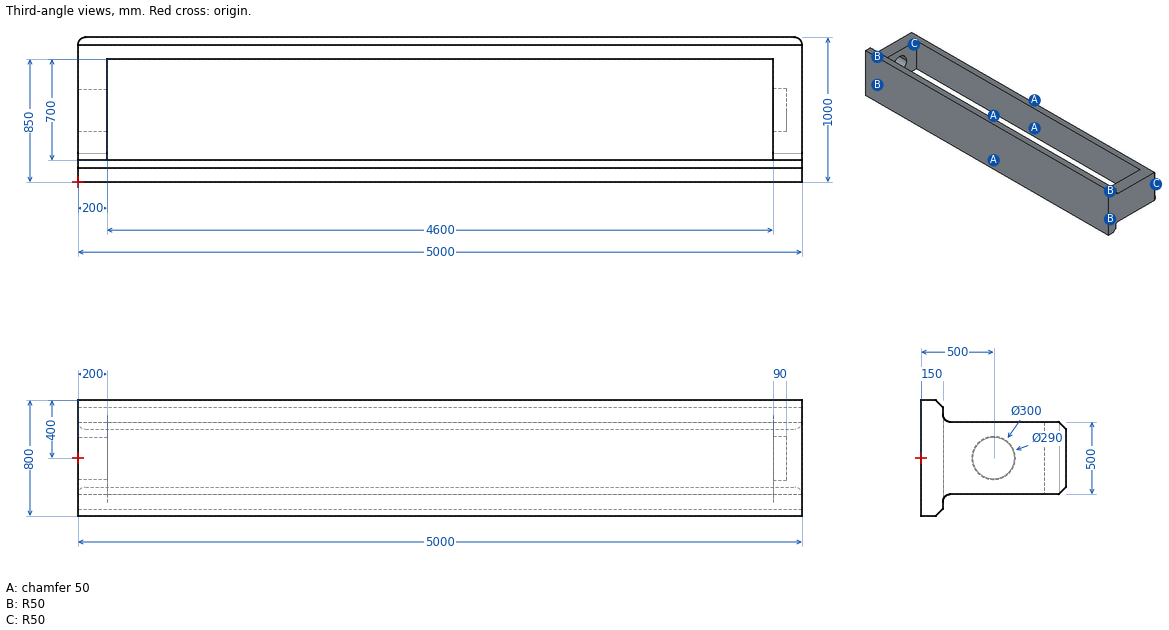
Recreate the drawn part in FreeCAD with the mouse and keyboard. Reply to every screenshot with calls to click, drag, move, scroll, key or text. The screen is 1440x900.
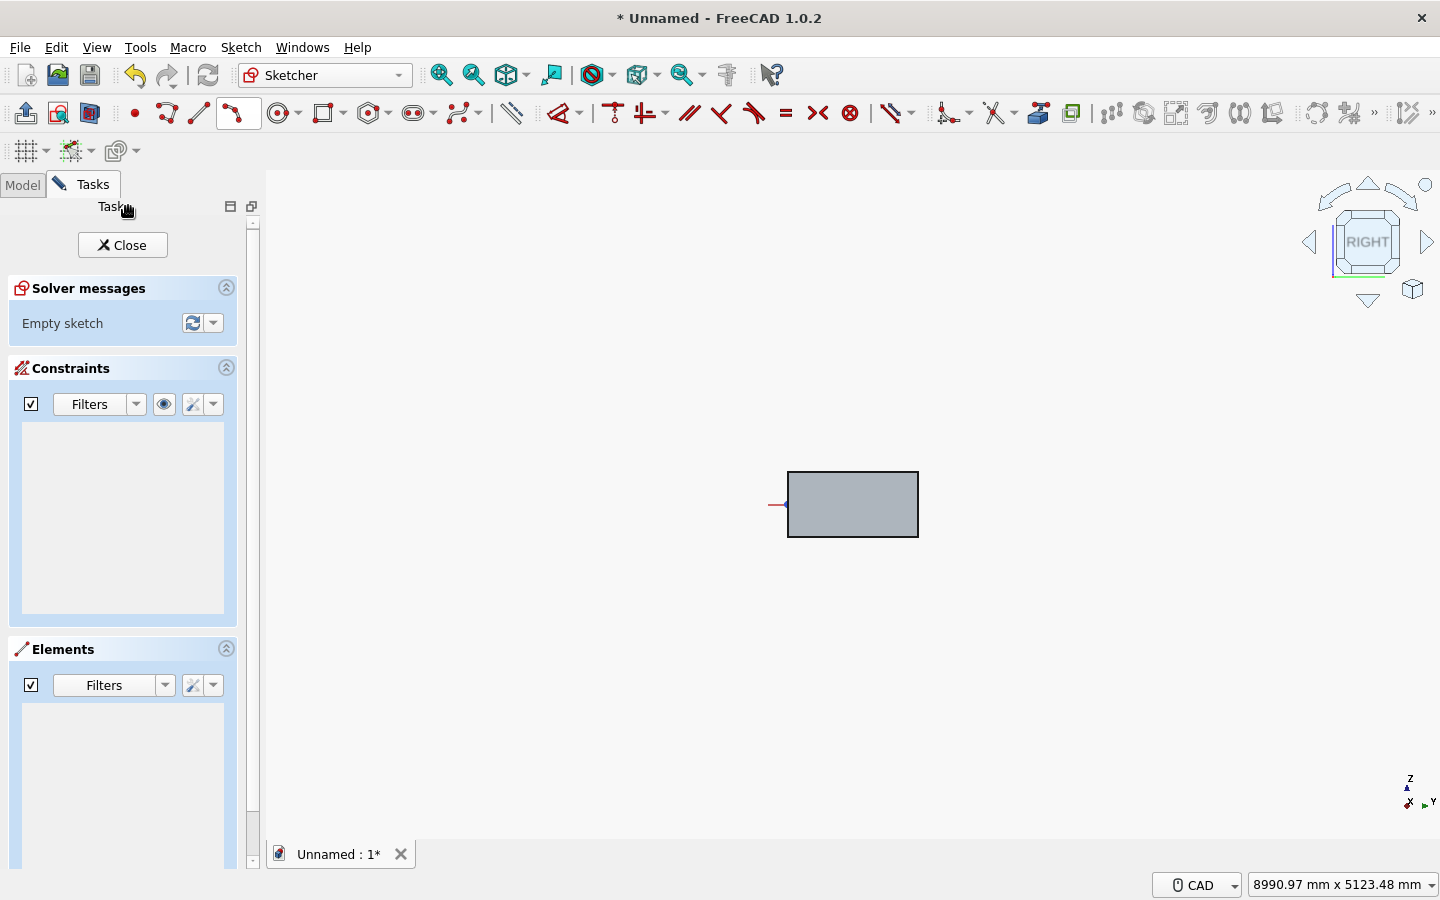
key(q)
key(s)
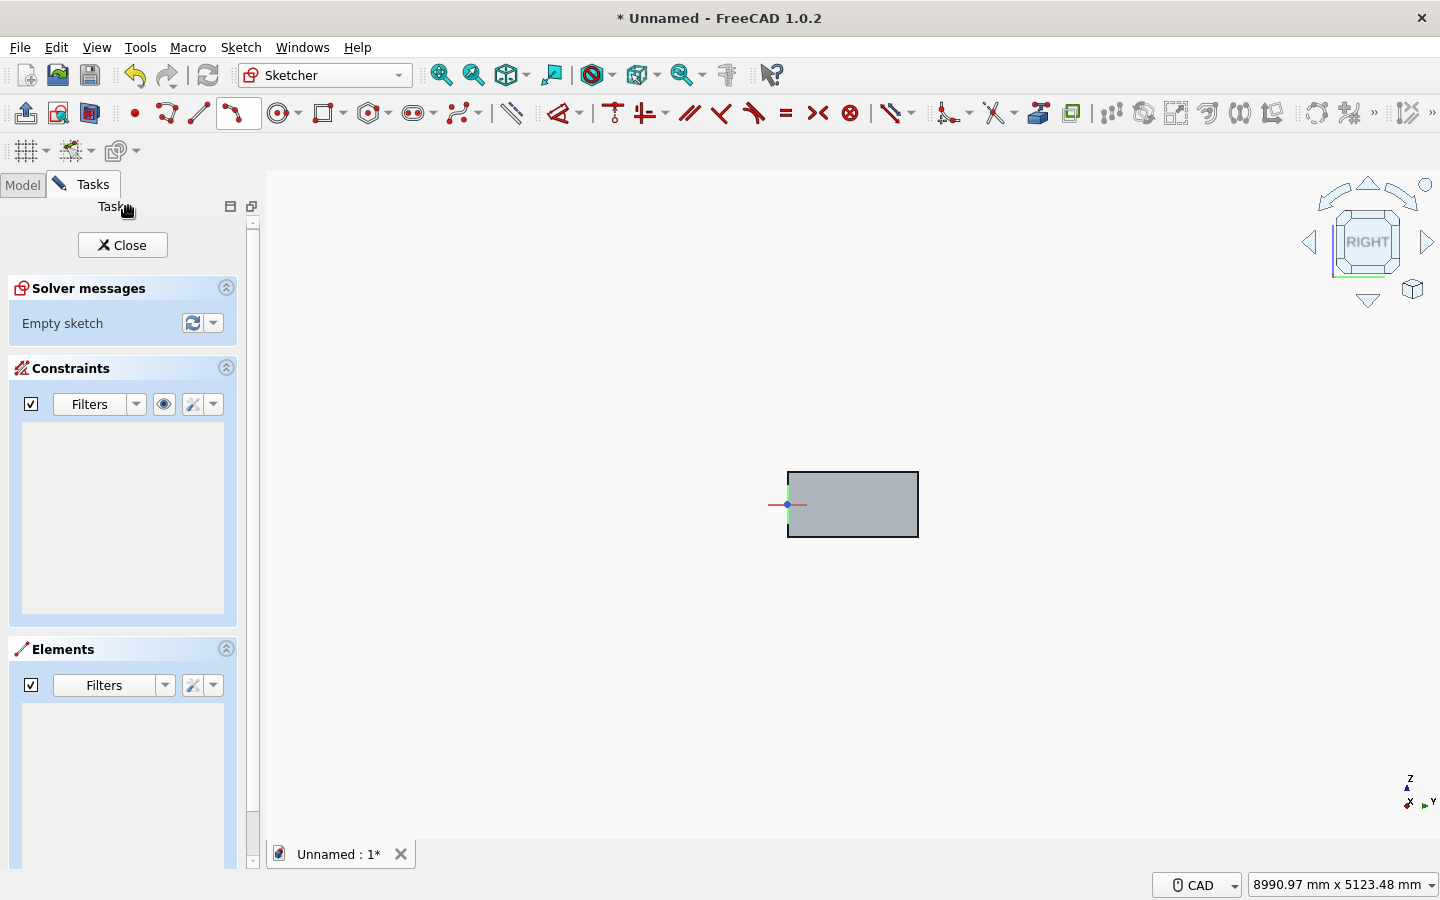
scroll(835, 504, up, 11)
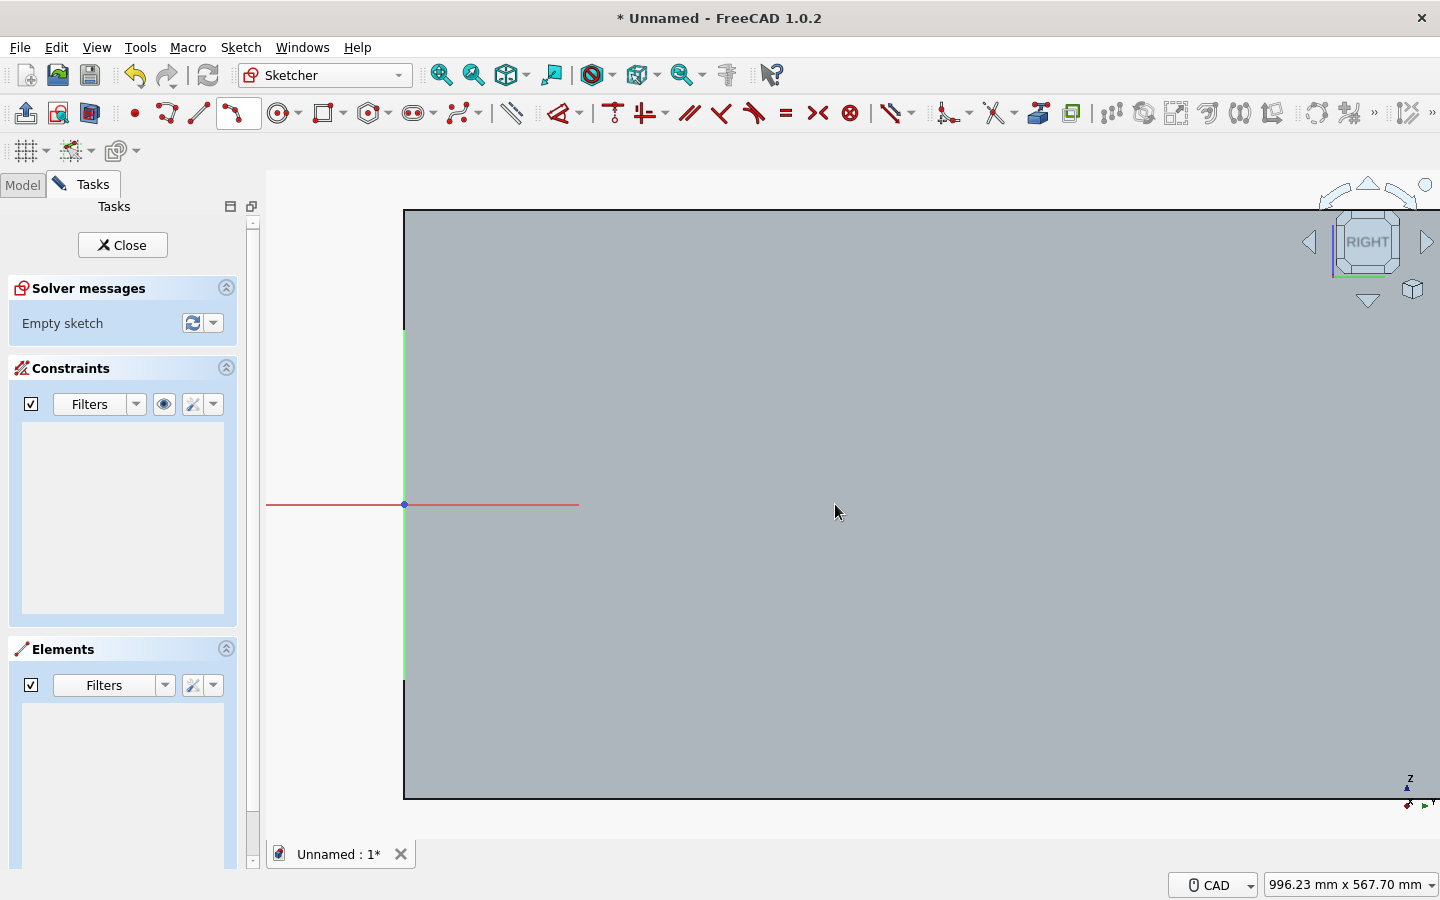
key(g)
key(c)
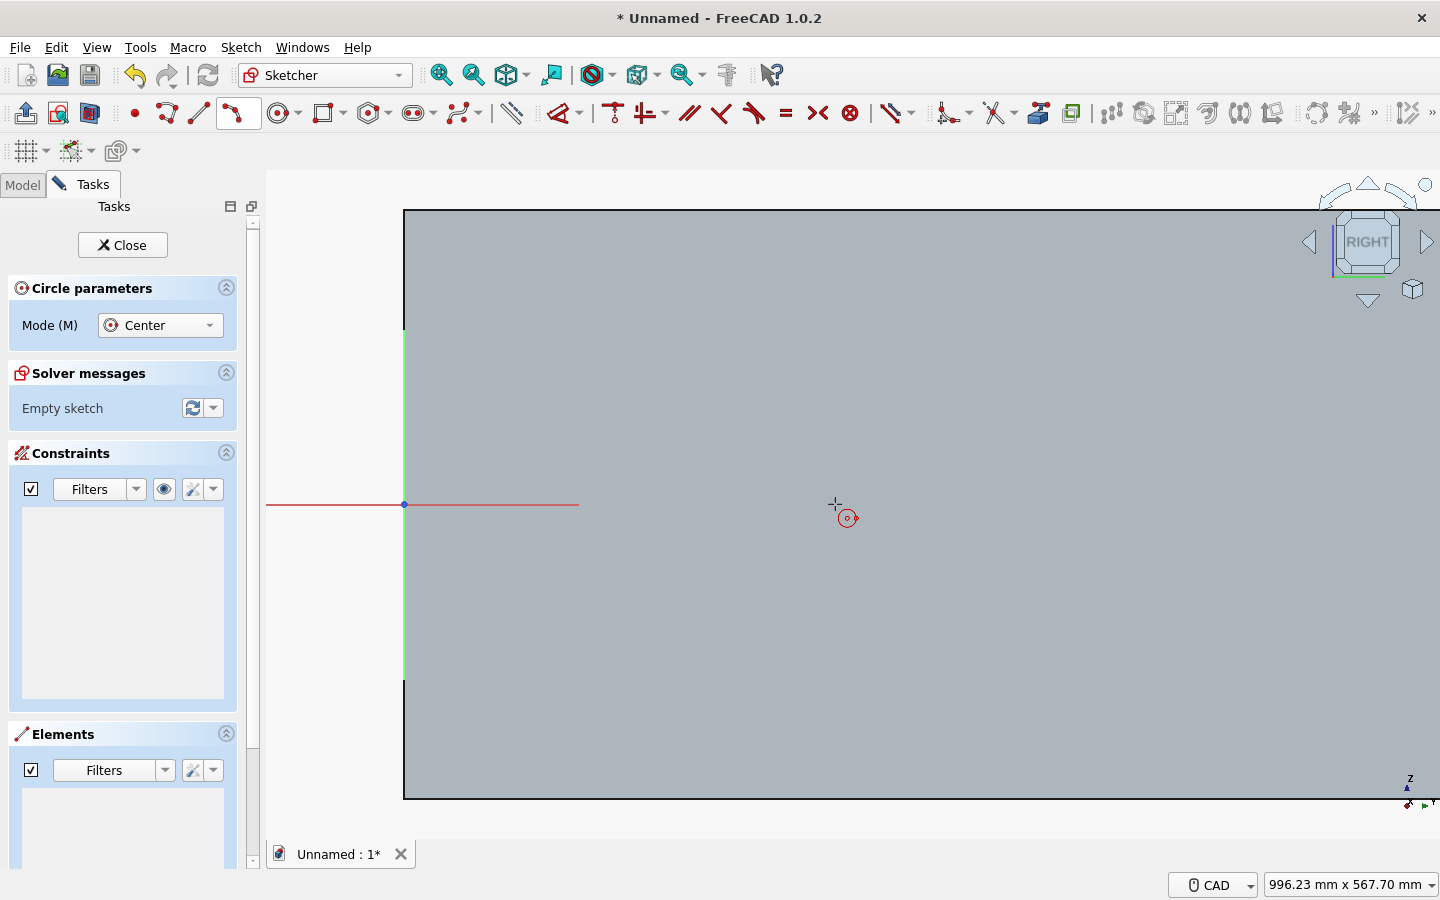
click(994, 504)
click(1114, 384)
key(Escape)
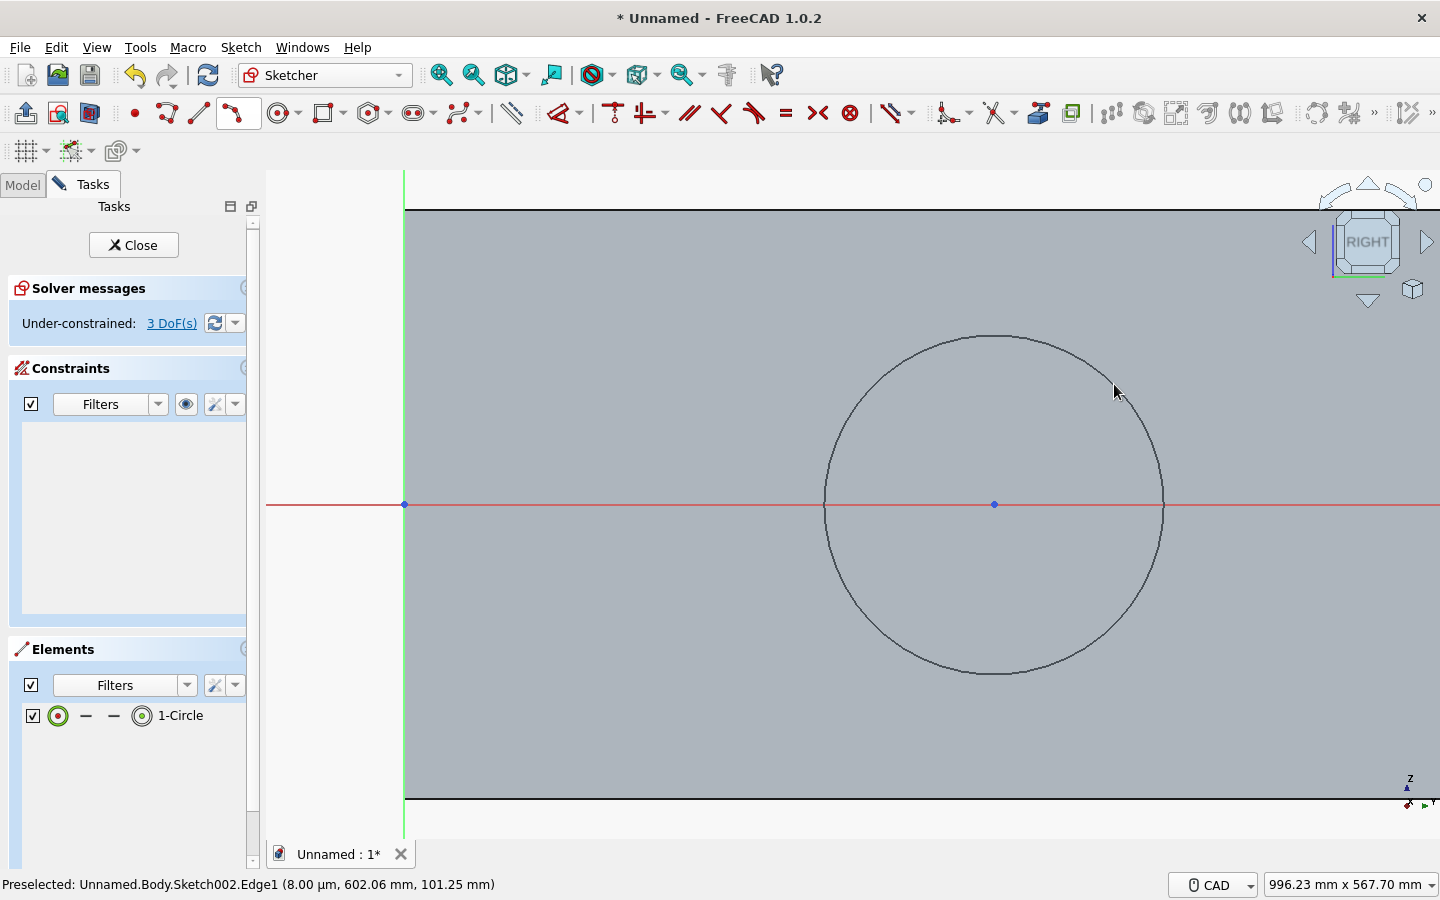
click(994, 505)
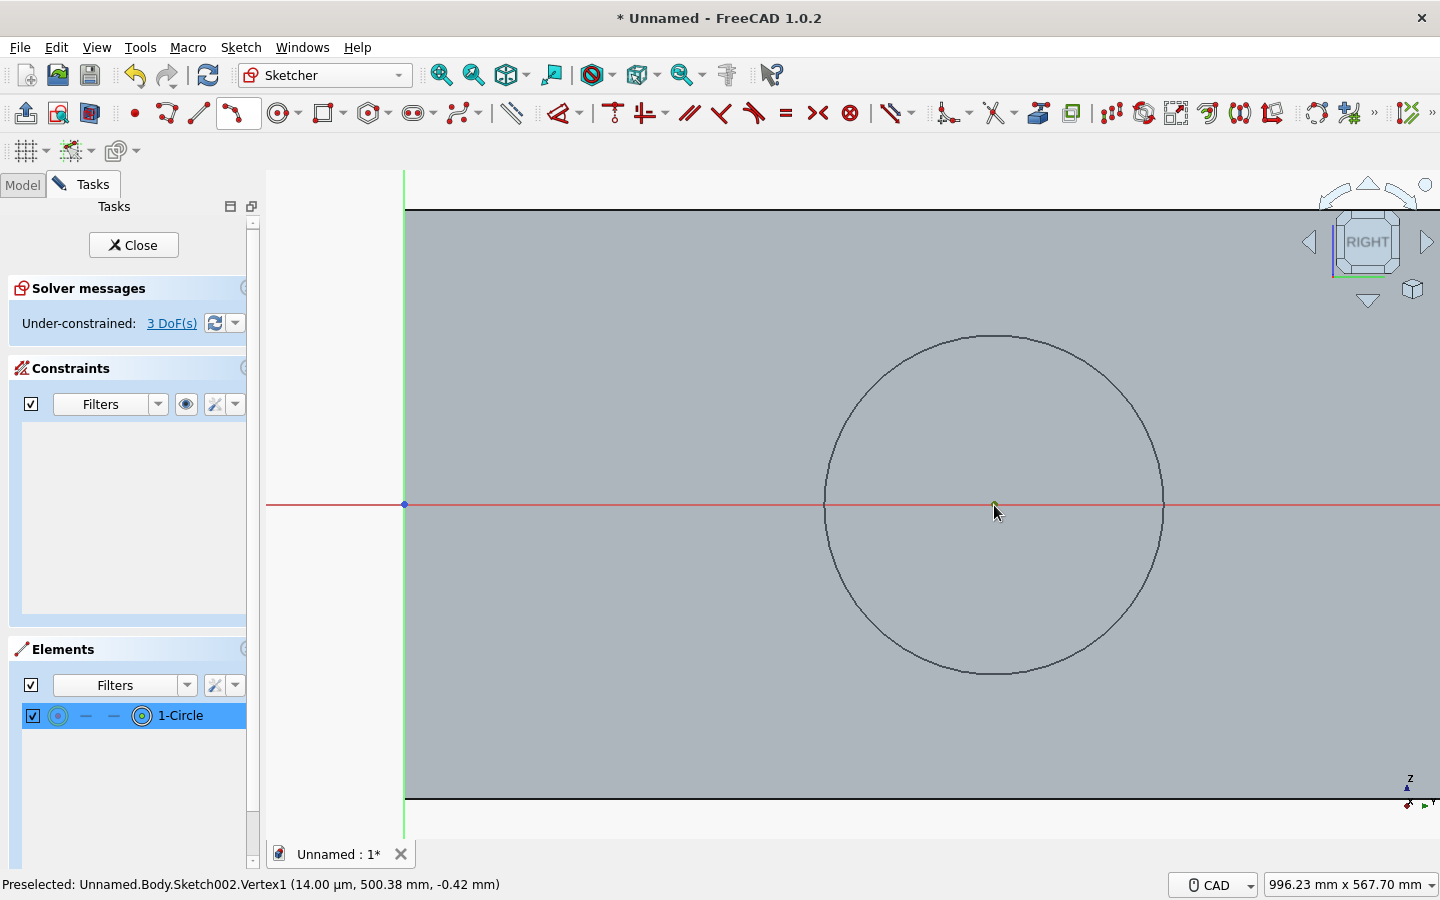
click(364, 504)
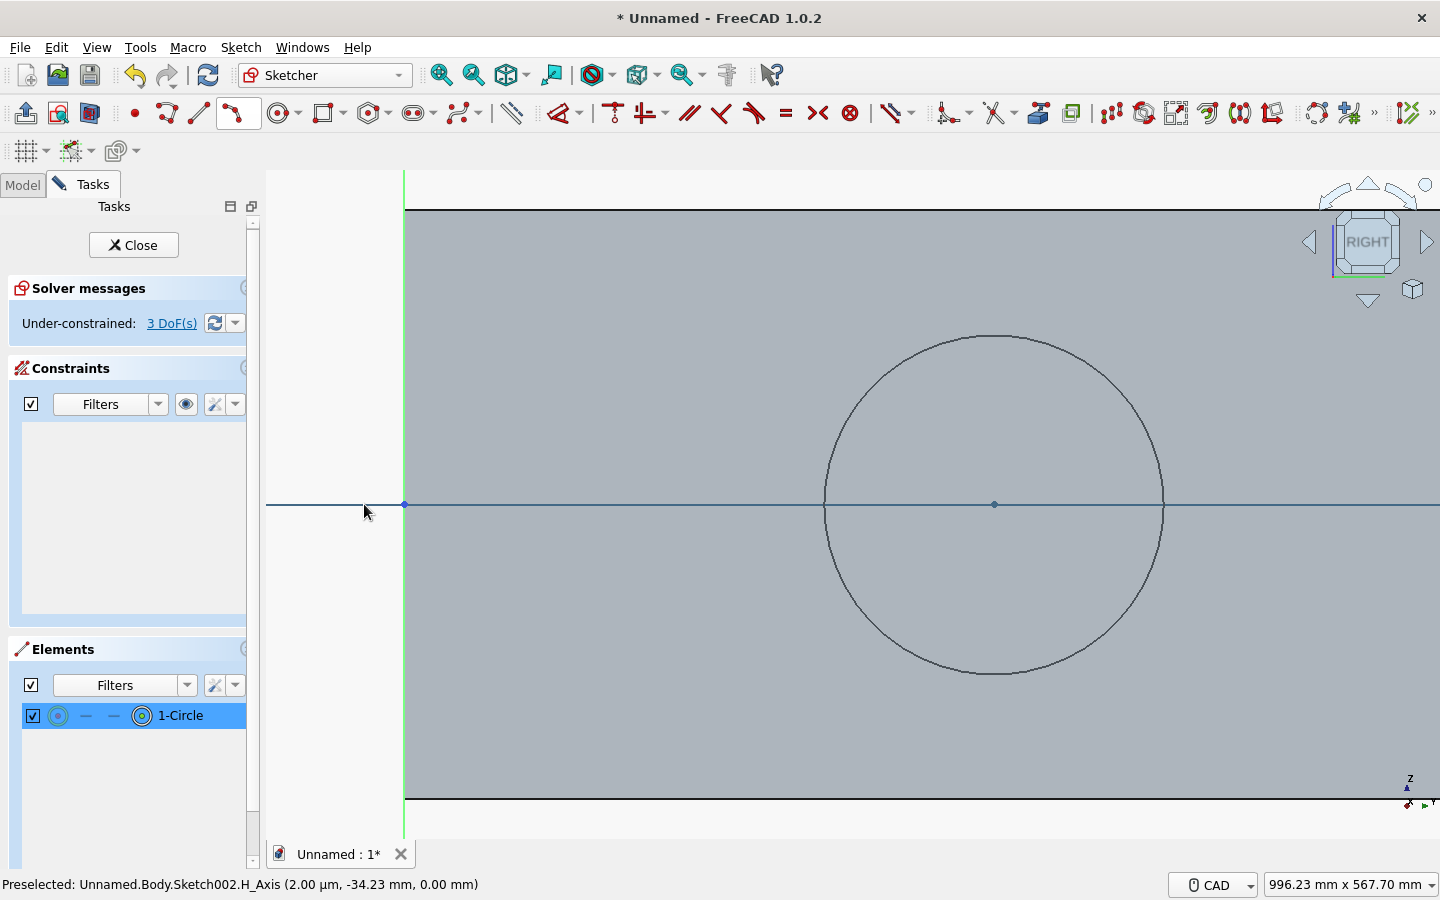
key(c)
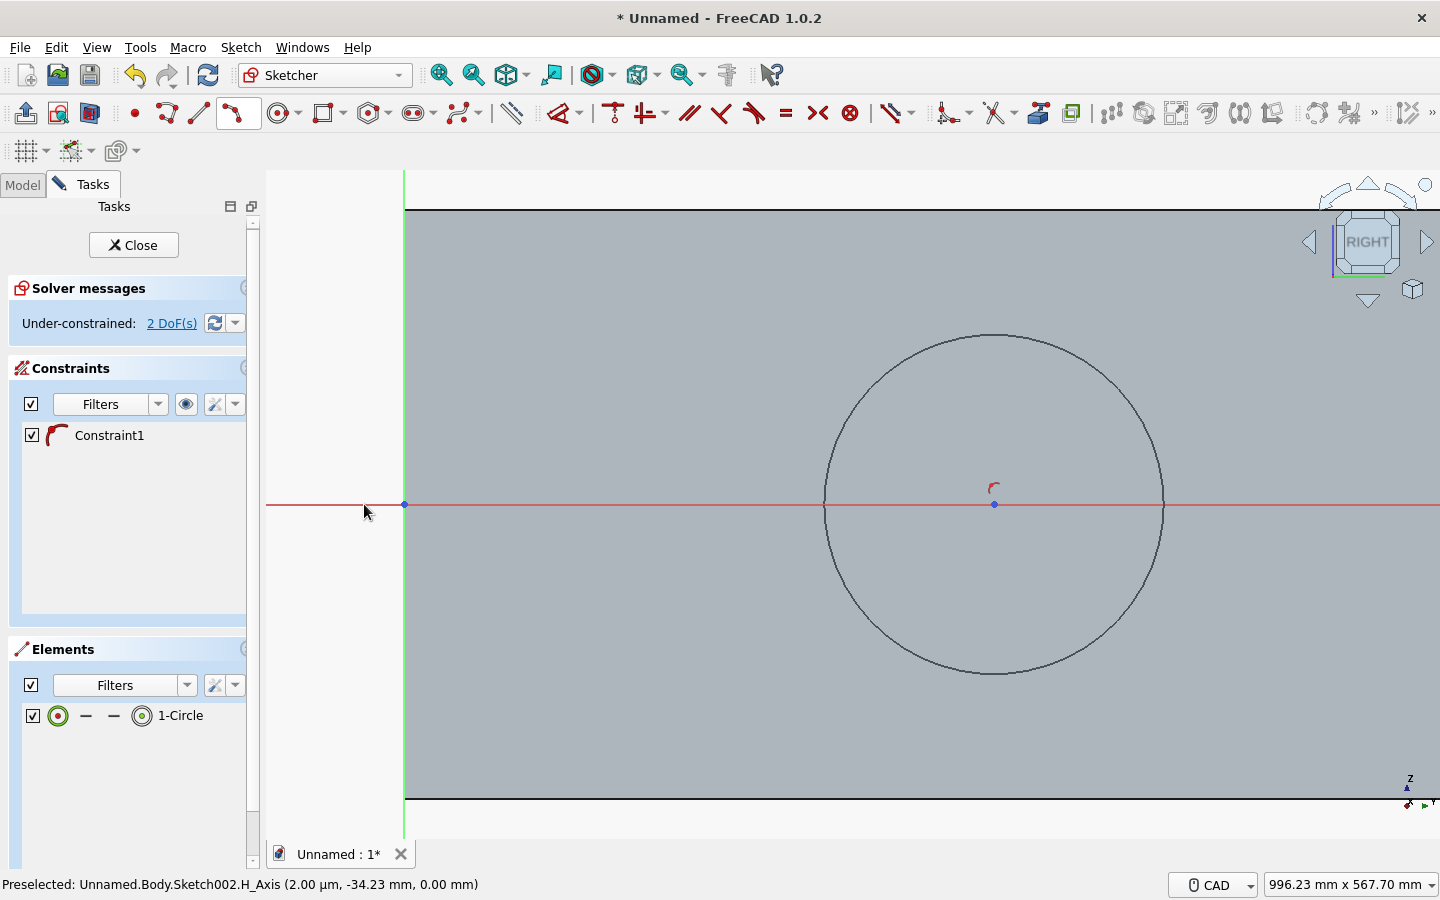
key(d)